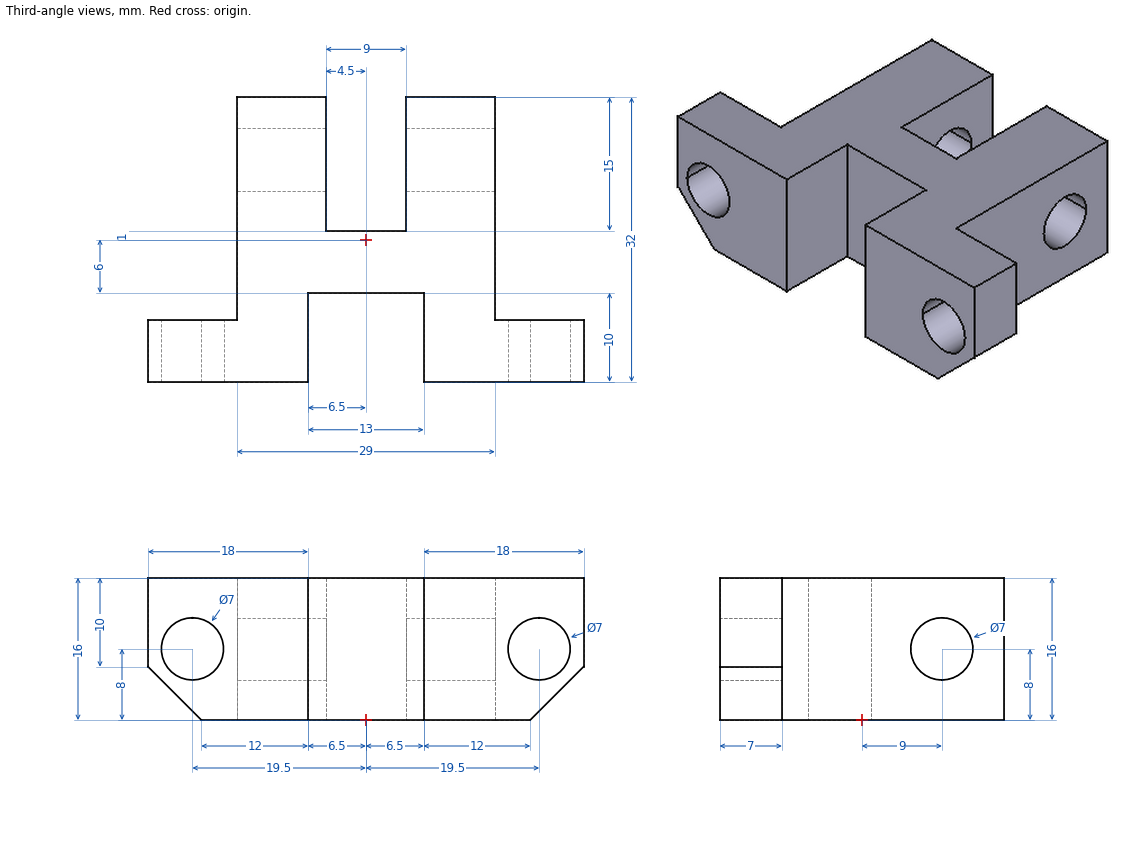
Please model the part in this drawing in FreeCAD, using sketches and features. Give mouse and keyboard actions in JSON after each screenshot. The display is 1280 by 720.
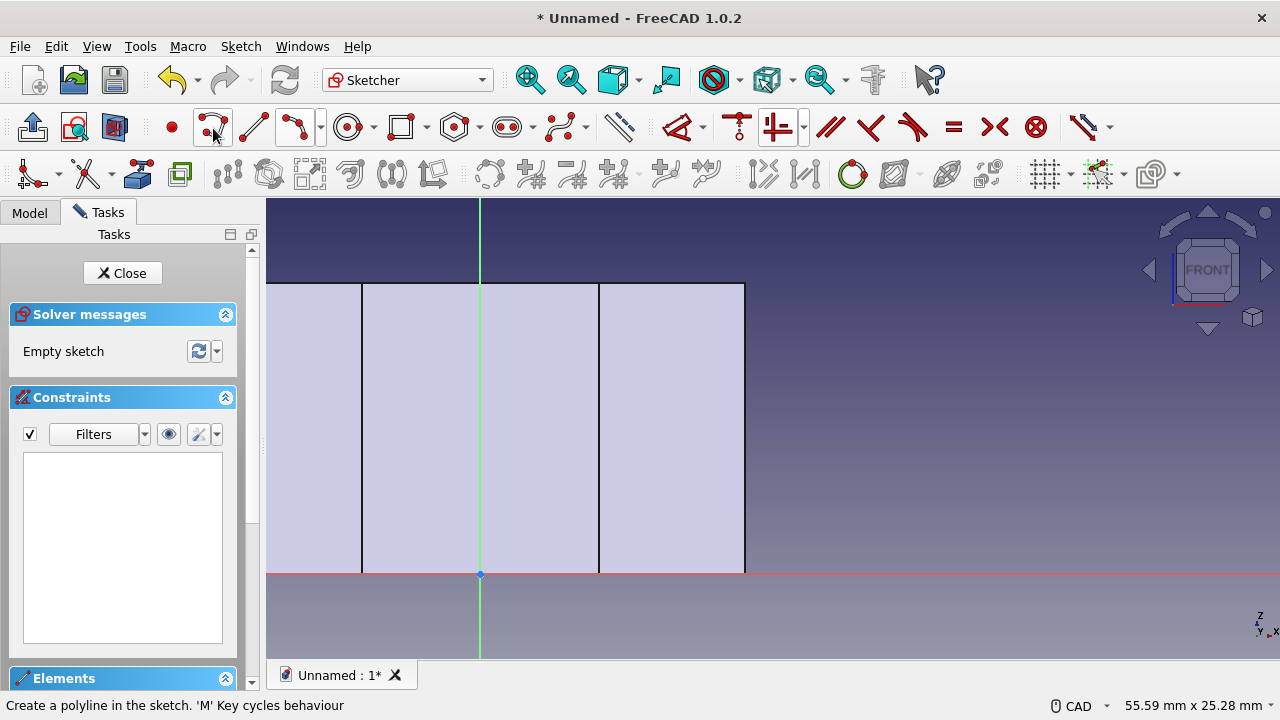
{"action": "left_click", "coordinate": [599, 574]}
{"action": "left_click", "coordinate": [818, 565]}
{"action": "left_click", "coordinate": [927, 465]}
{"action": "left_click", "coordinate": [927, 283]}
{"action": "left_click", "coordinate": [599, 283]}
{"action": "left_click", "coordinate": [599, 574]}
{"action": "key", "text": "Escape"}
{"action": "key", "text": "Escape"}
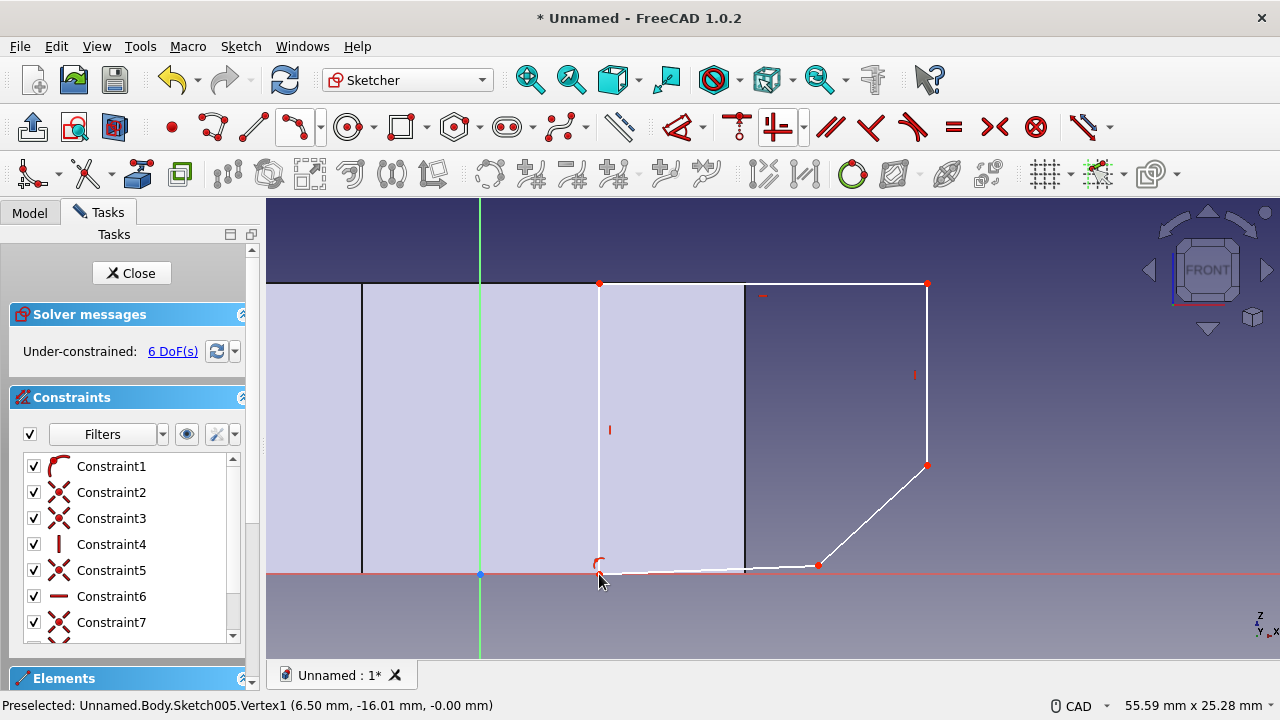
{"action": "left_click", "coordinate": [665, 572]}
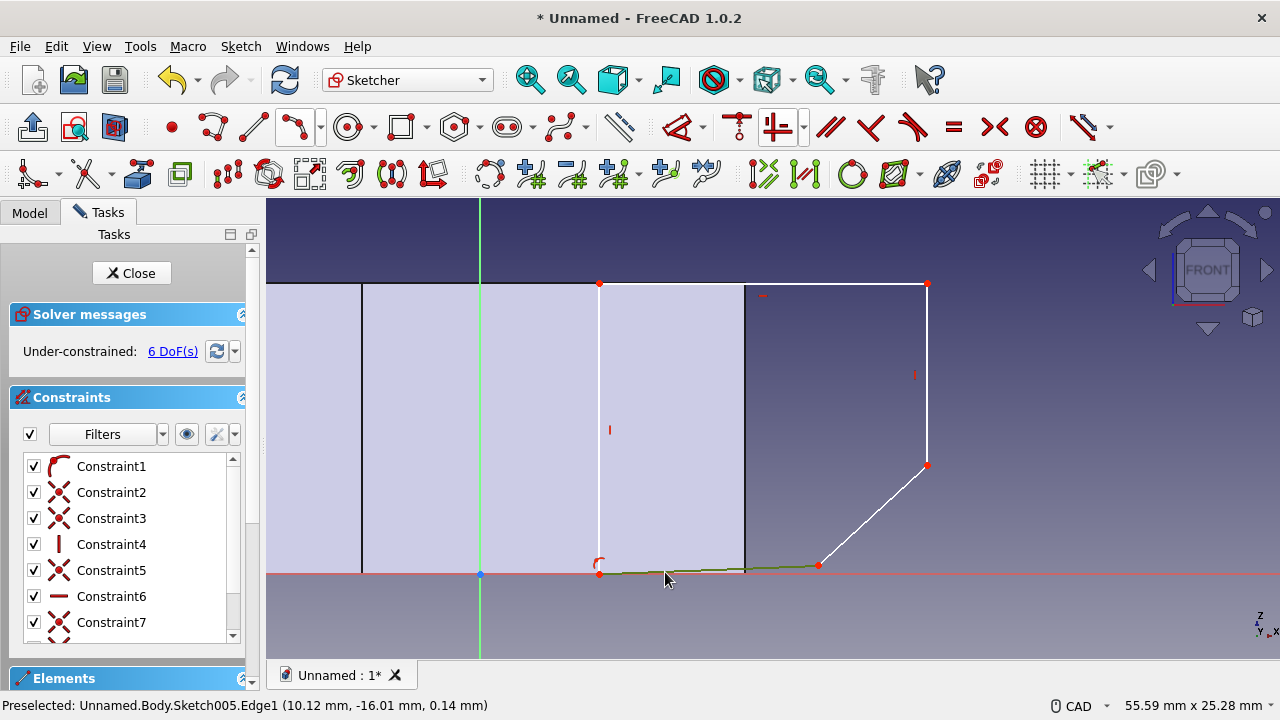
{"action": "left_click", "coordinate": [804, 128]}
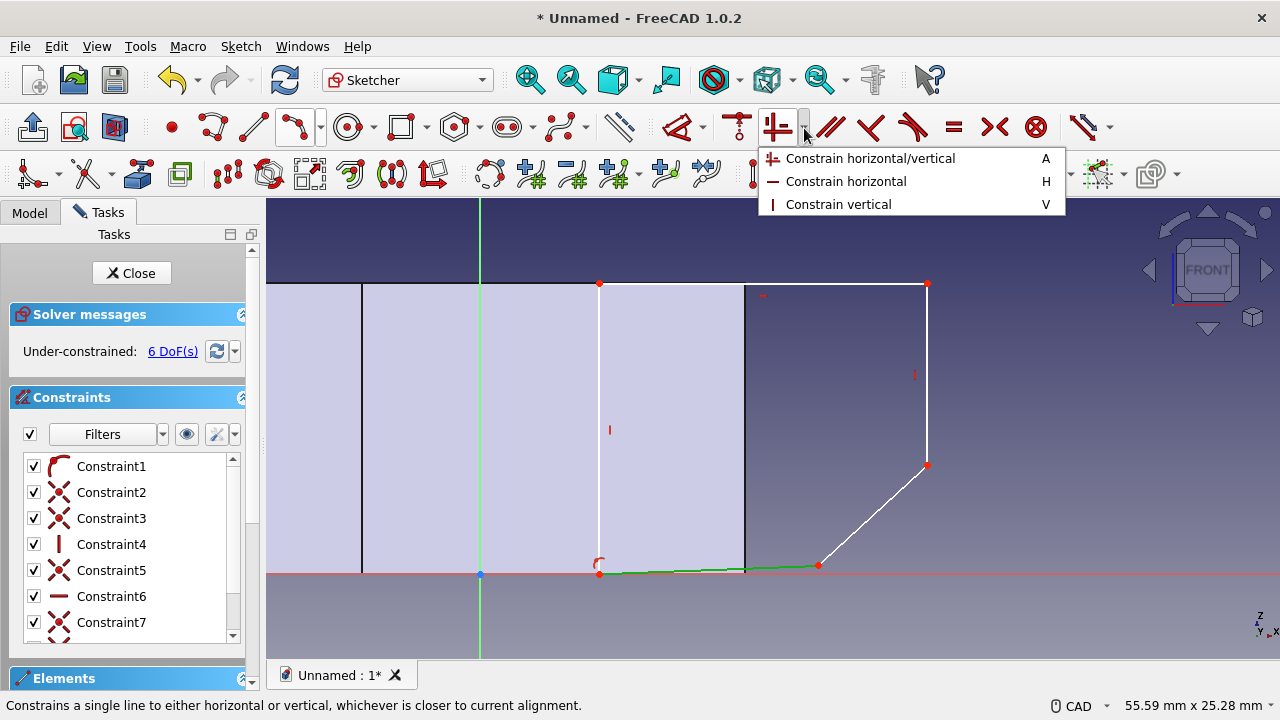
{"action": "left_click", "coordinate": [912, 182]}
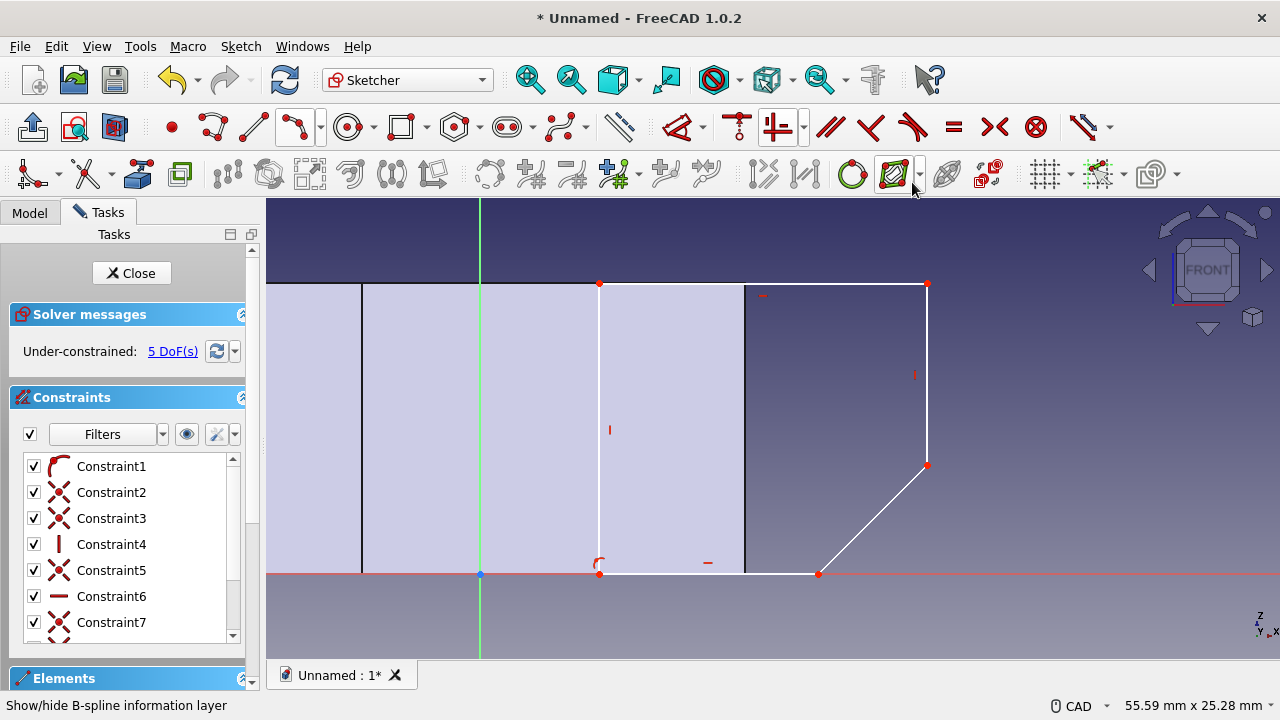
{"action": "left_click", "coordinate": [676, 128]}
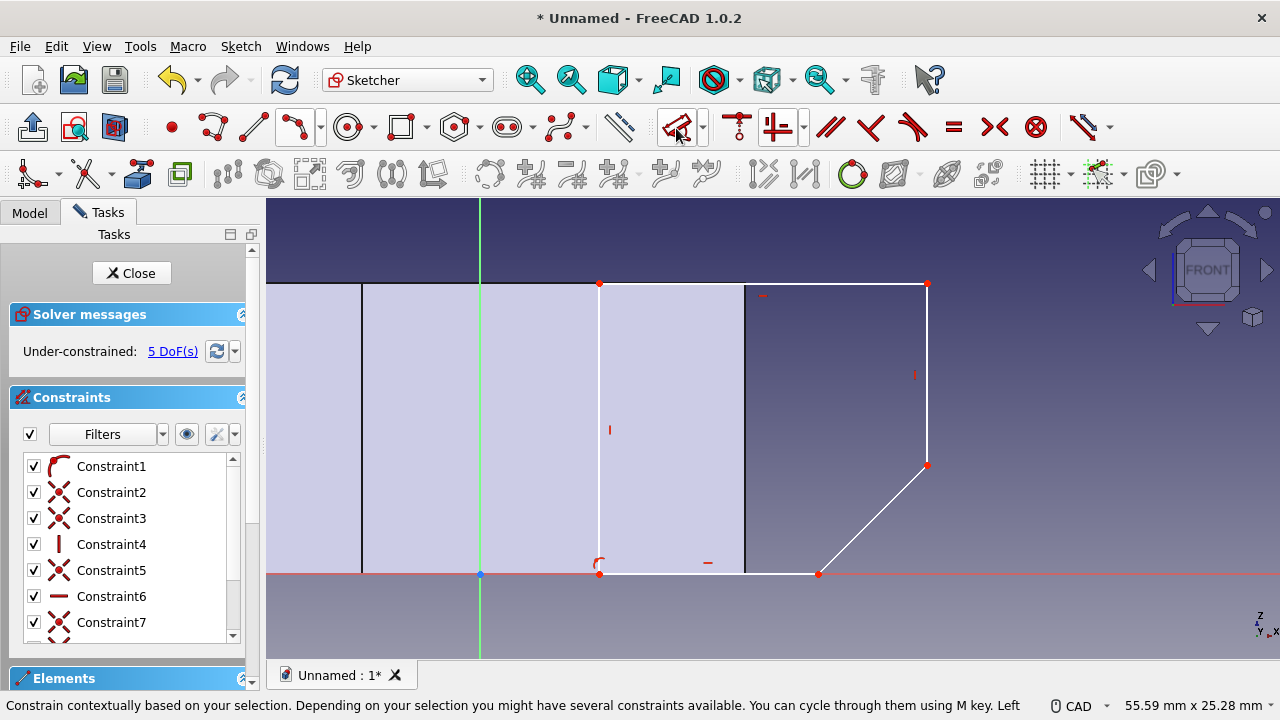
{"action": "left_click", "coordinate": [665, 574]}
{"action": "left_click", "coordinate": [709, 608]}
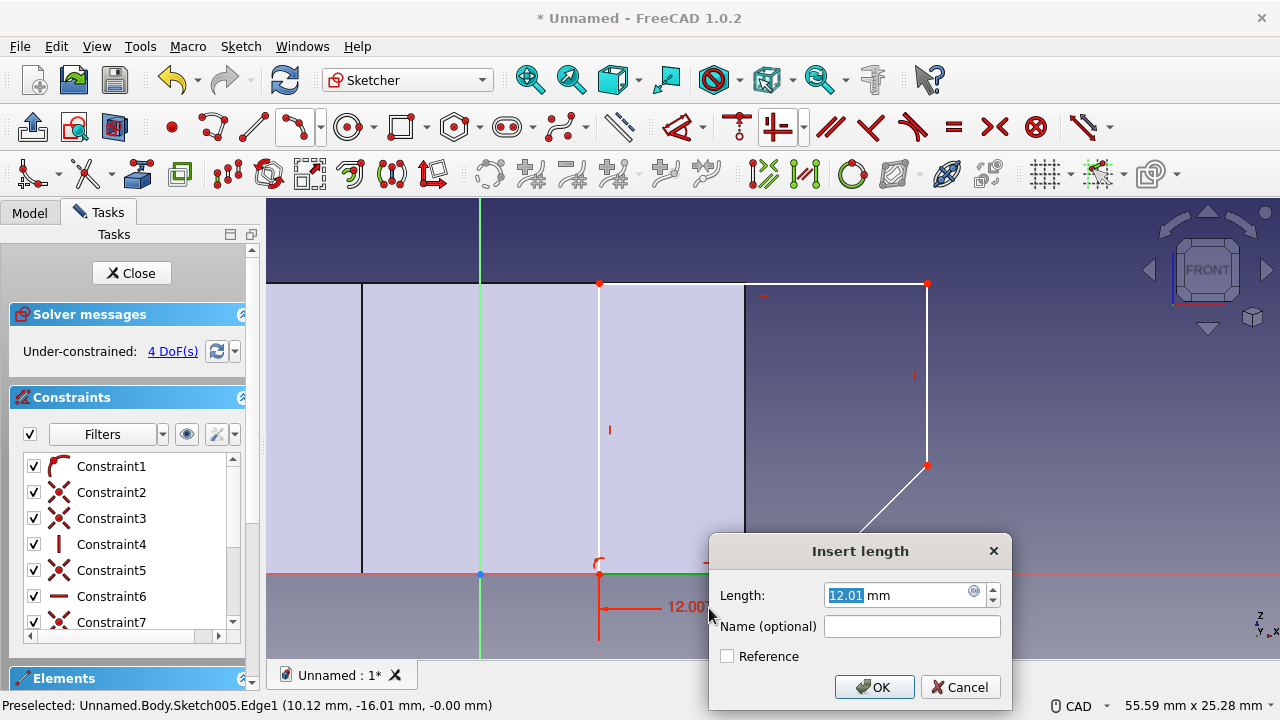
{"action": "type", "text": "12"}
{"action": "key", "text": "Return"}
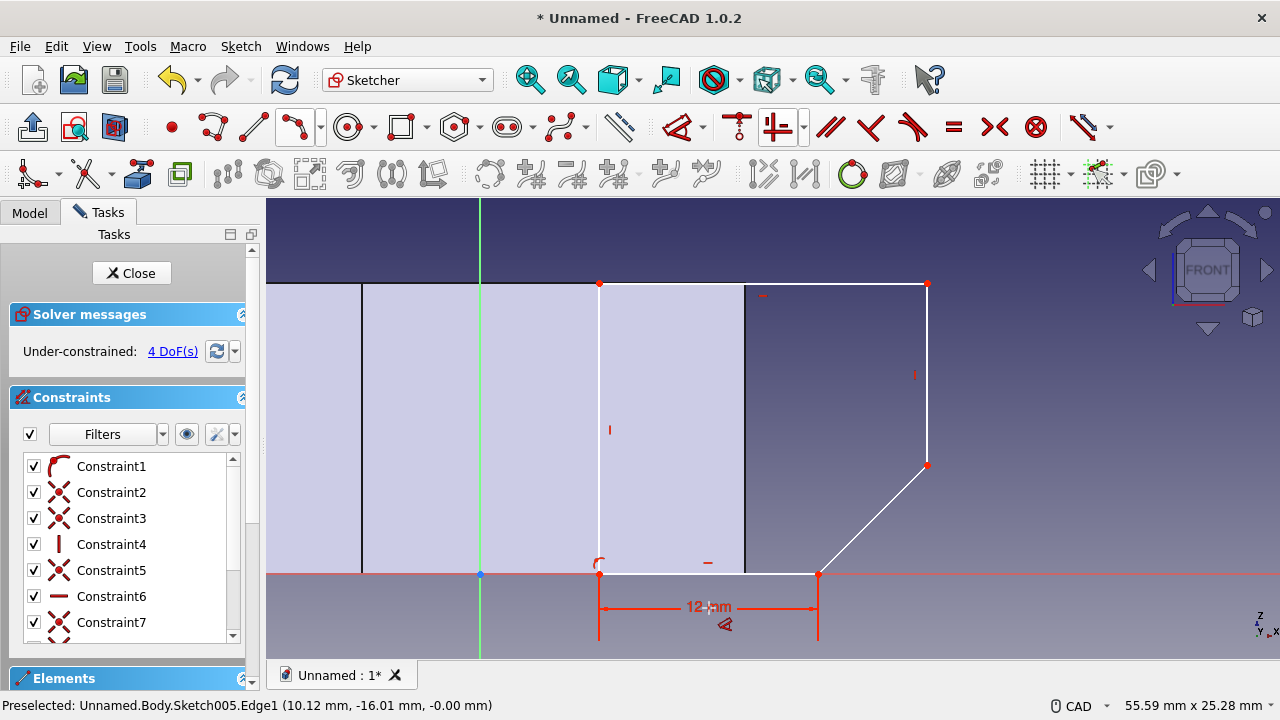
{"action": "left_click", "coordinate": [927, 411]}
{"action": "left_click", "coordinate": [961, 375]}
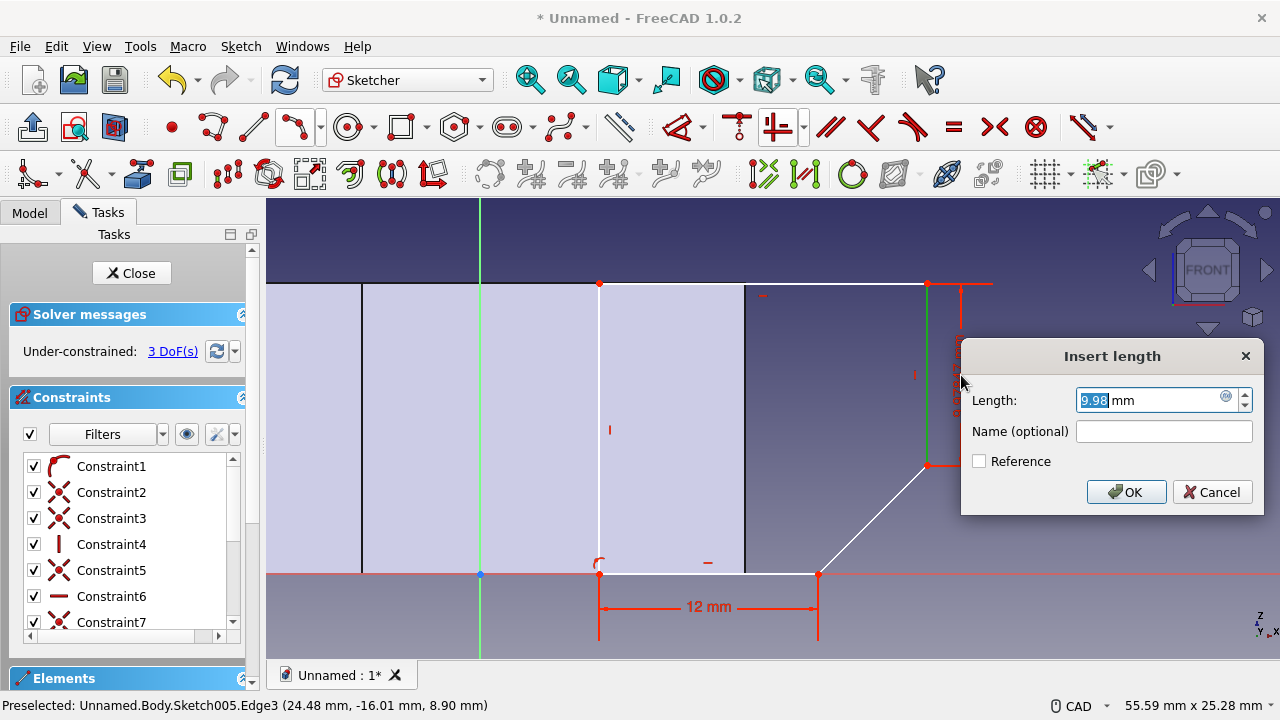
{"action": "type", "text": "10"}
{"action": "key", "text": "Return"}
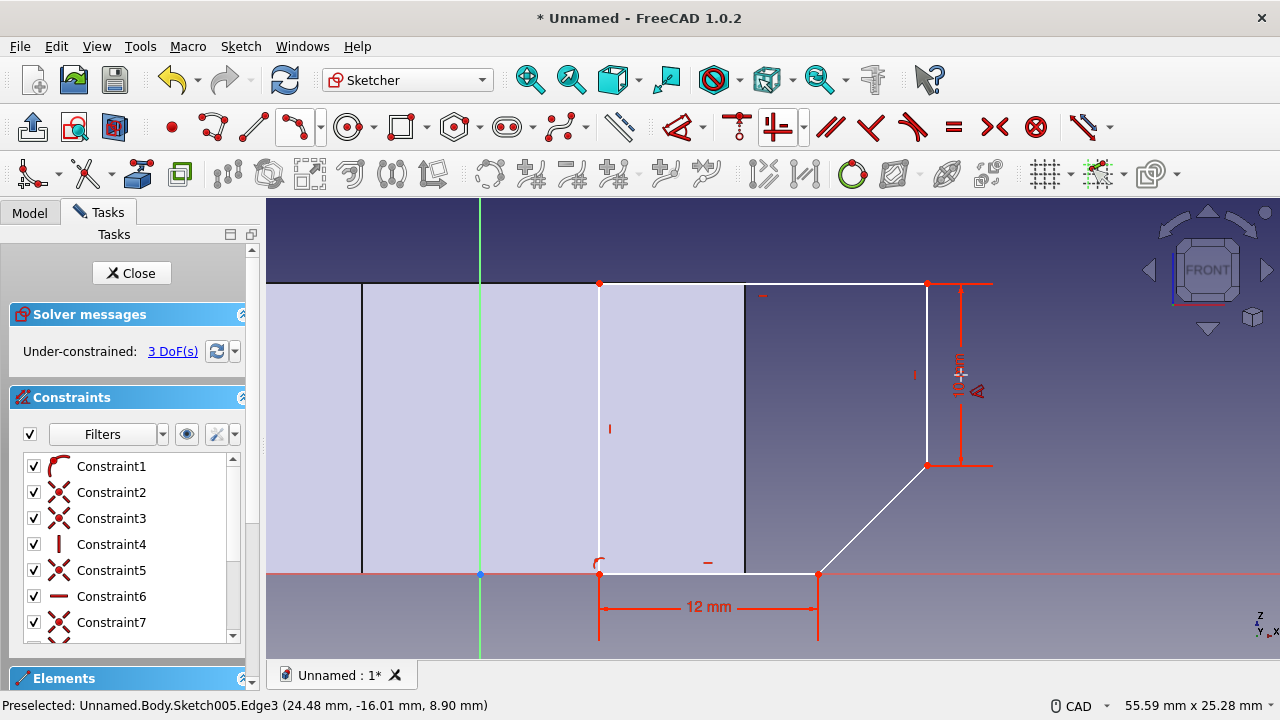
{"action": "left_click", "coordinate": [829, 284]}
{"action": "left_click", "coordinate": [763, 250]}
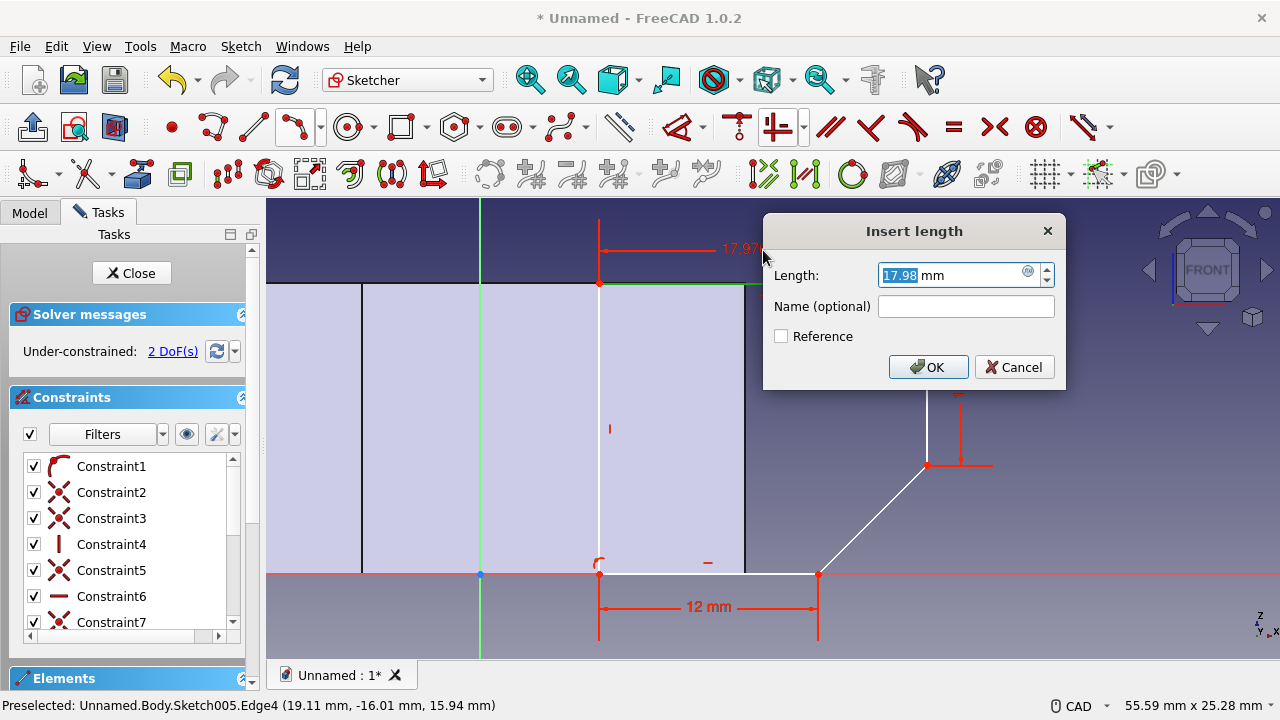
{"action": "type", "text": "18"}
{"action": "key", "text": "Return"}